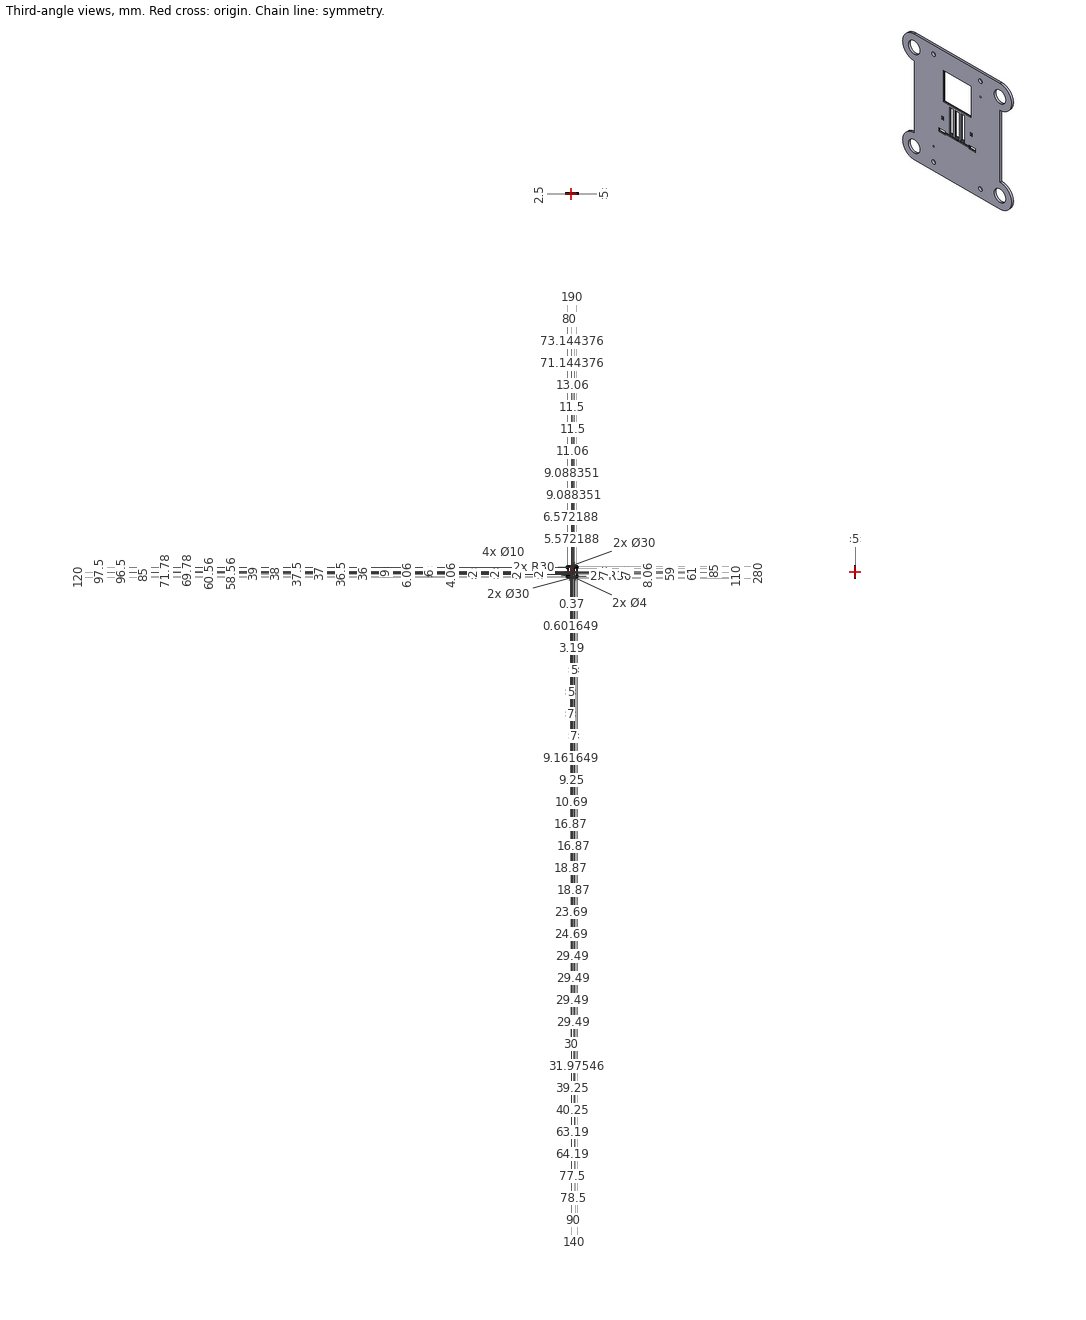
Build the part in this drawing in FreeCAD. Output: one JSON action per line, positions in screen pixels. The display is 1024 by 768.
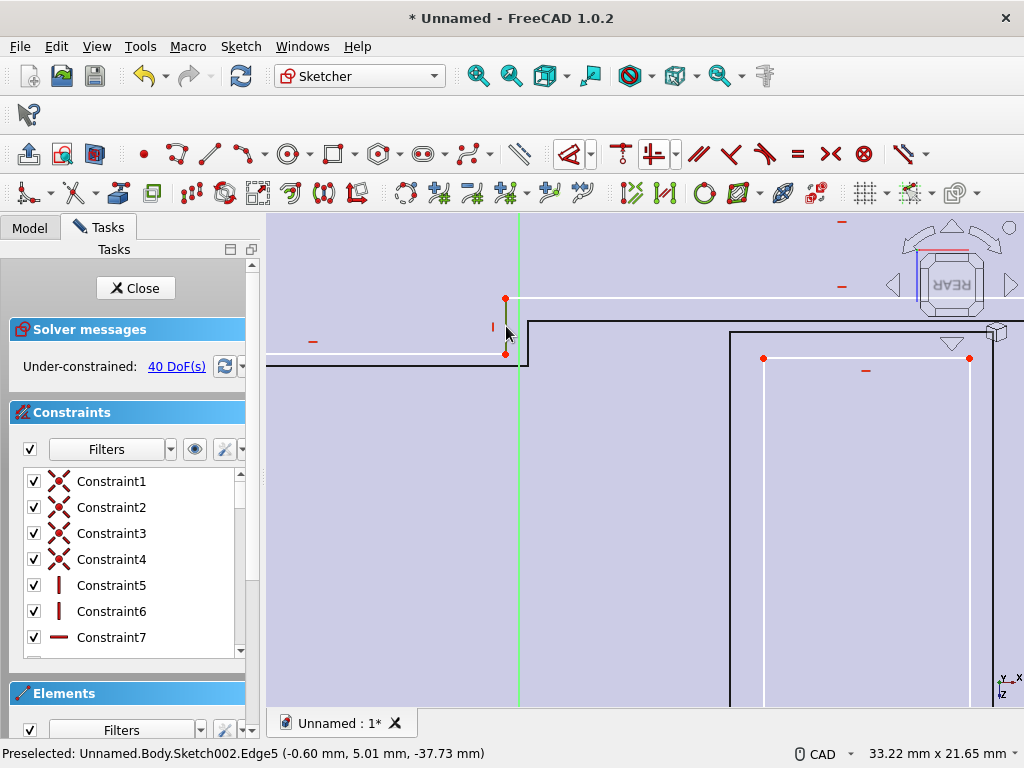
{"action": "key", "text": "i"}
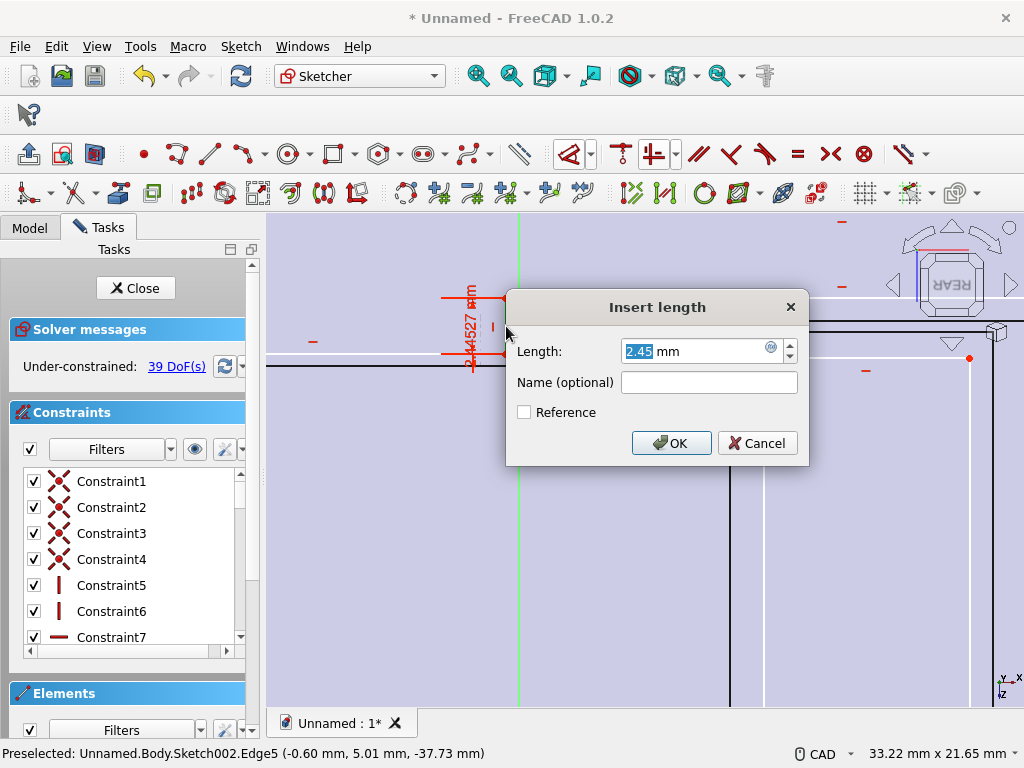
{"action": "type", "text": "2"}
{"action": "key", "text": "Return"}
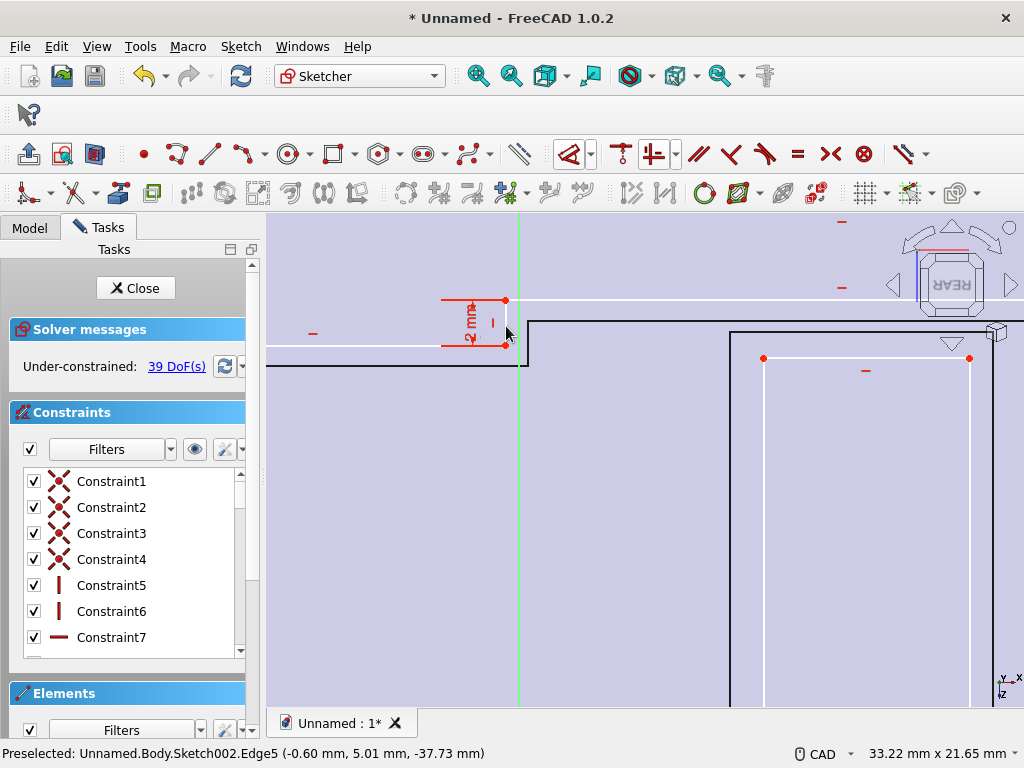
{"action": "scroll", "coordinate": [514, 329], "scroll_direction": "down", "scroll_amount": 12}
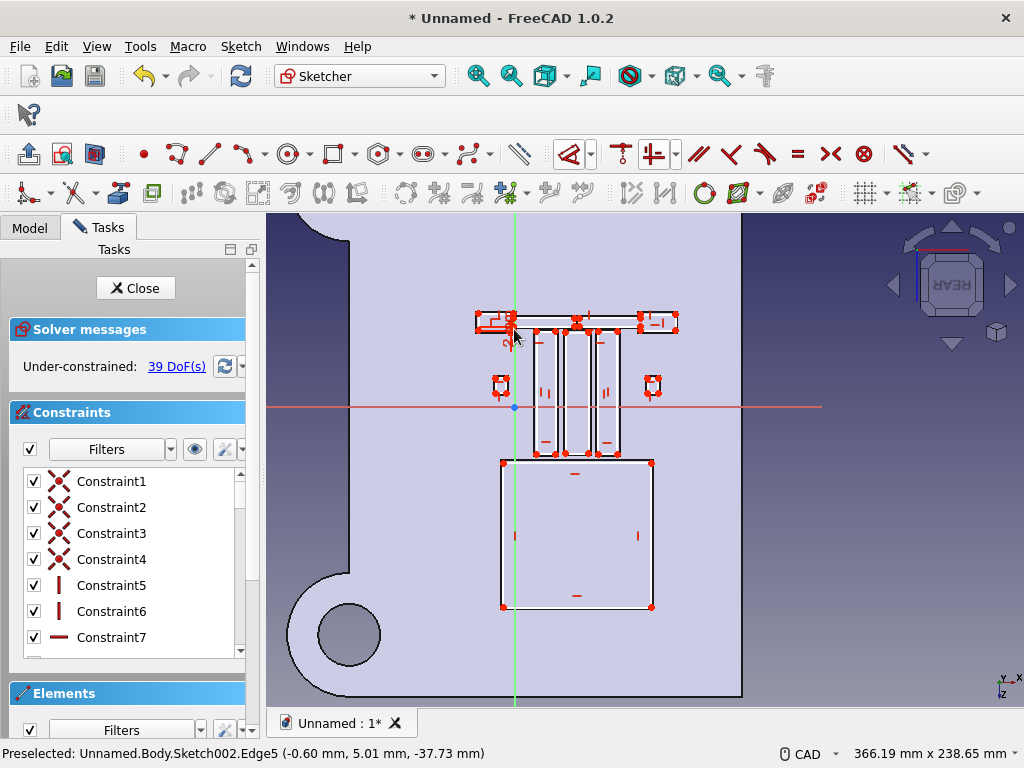
{"action": "scroll", "coordinate": [514, 317], "scroll_direction": "up", "scroll_amount": 13}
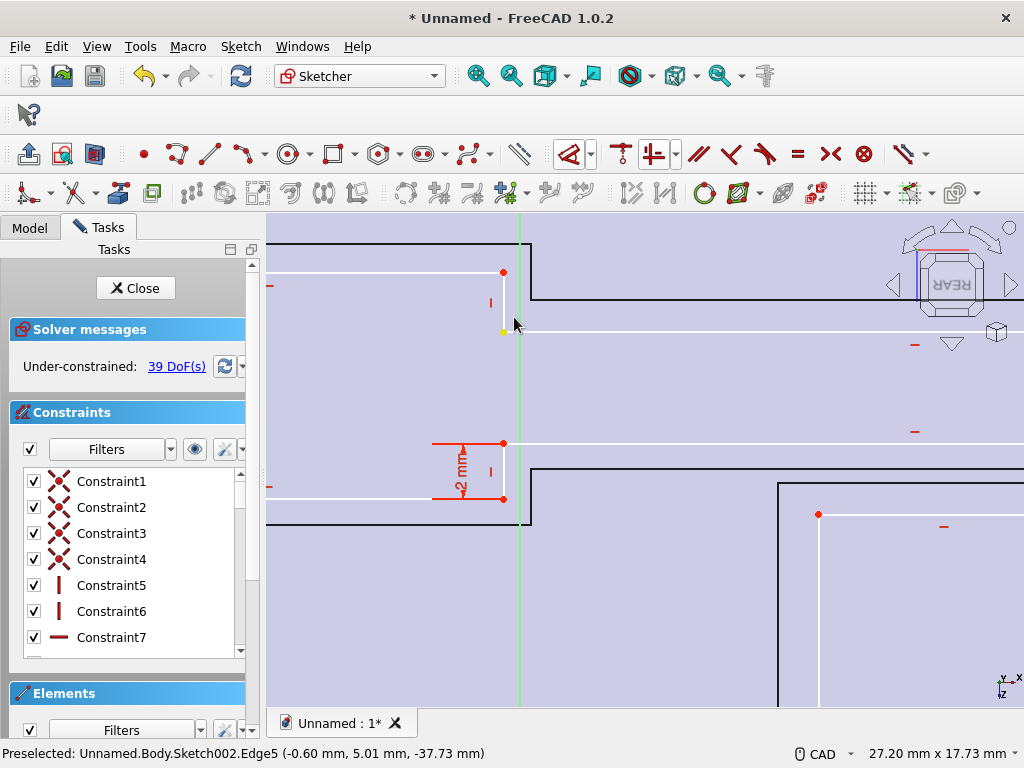
{"action": "left_click", "coordinate": [504, 314]}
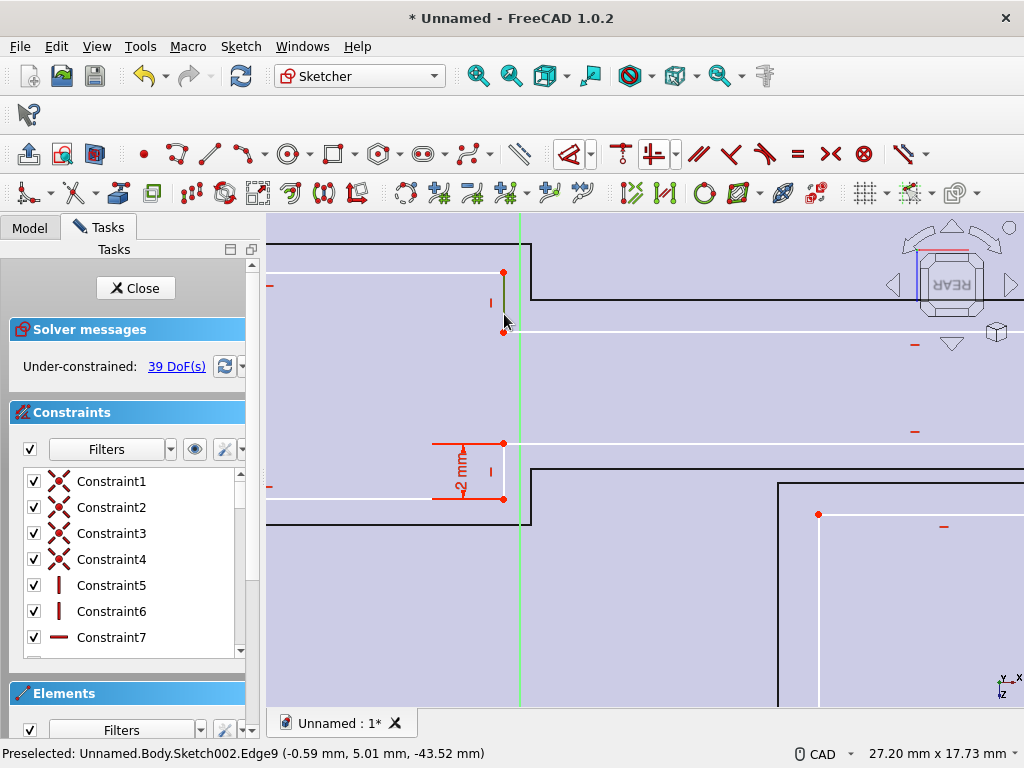
{"action": "left_click", "coordinate": [590, 154]}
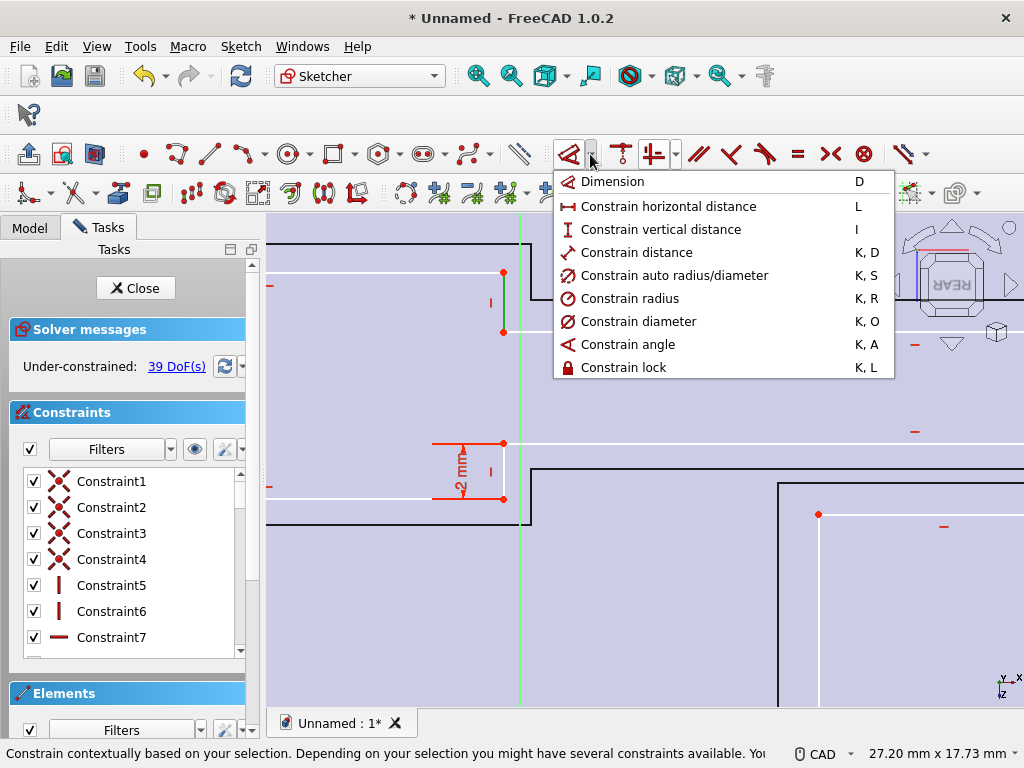
{"action": "left_click", "coordinate": [724, 230]}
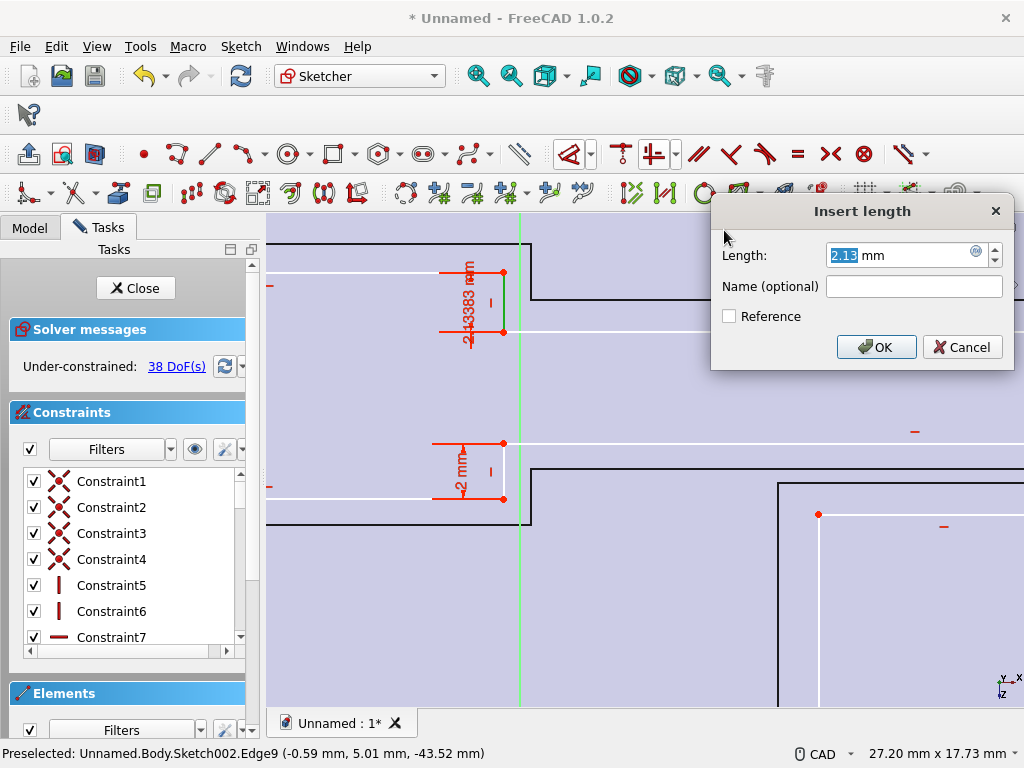
{"action": "type", "text": "2"}
{"action": "key", "text": "Return"}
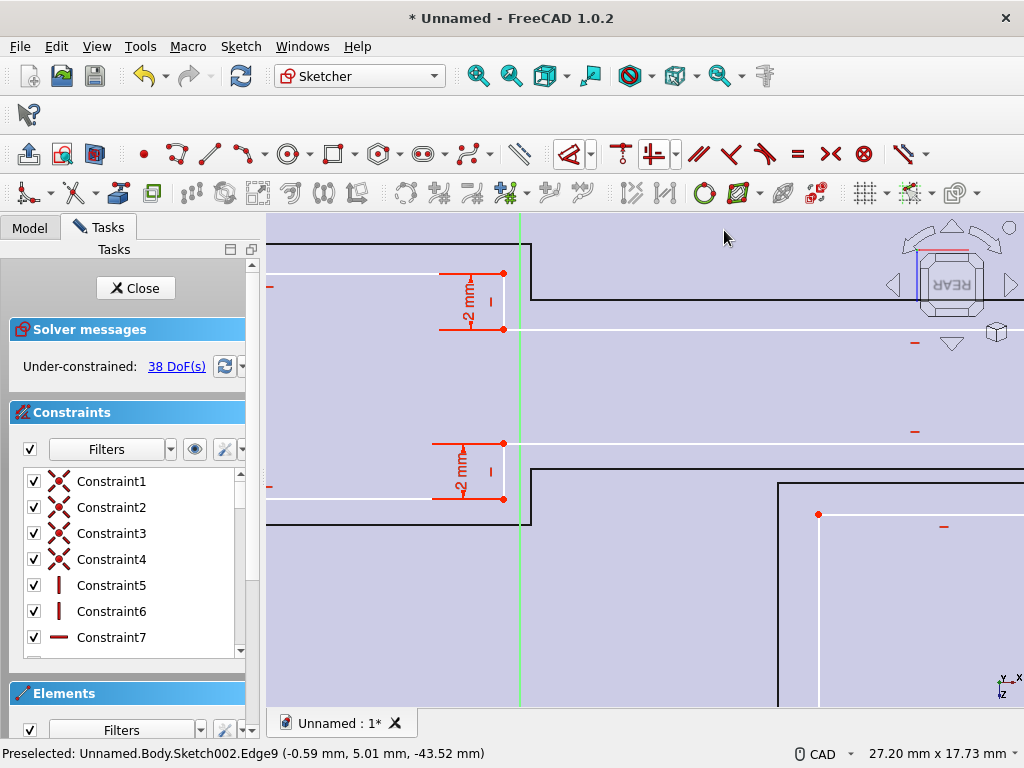
{"action": "scroll", "coordinate": [514, 317], "scroll_direction": "down", "scroll_amount": 13}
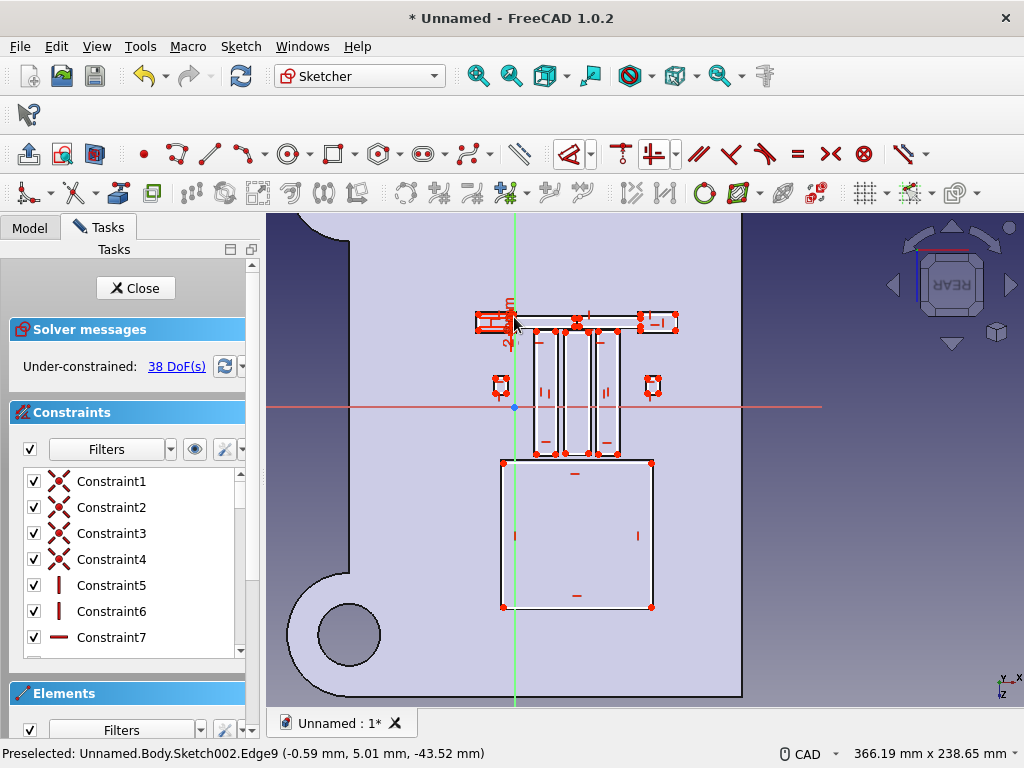
{"action": "scroll", "coordinate": [640, 328], "scroll_direction": "up", "scroll_amount": 13}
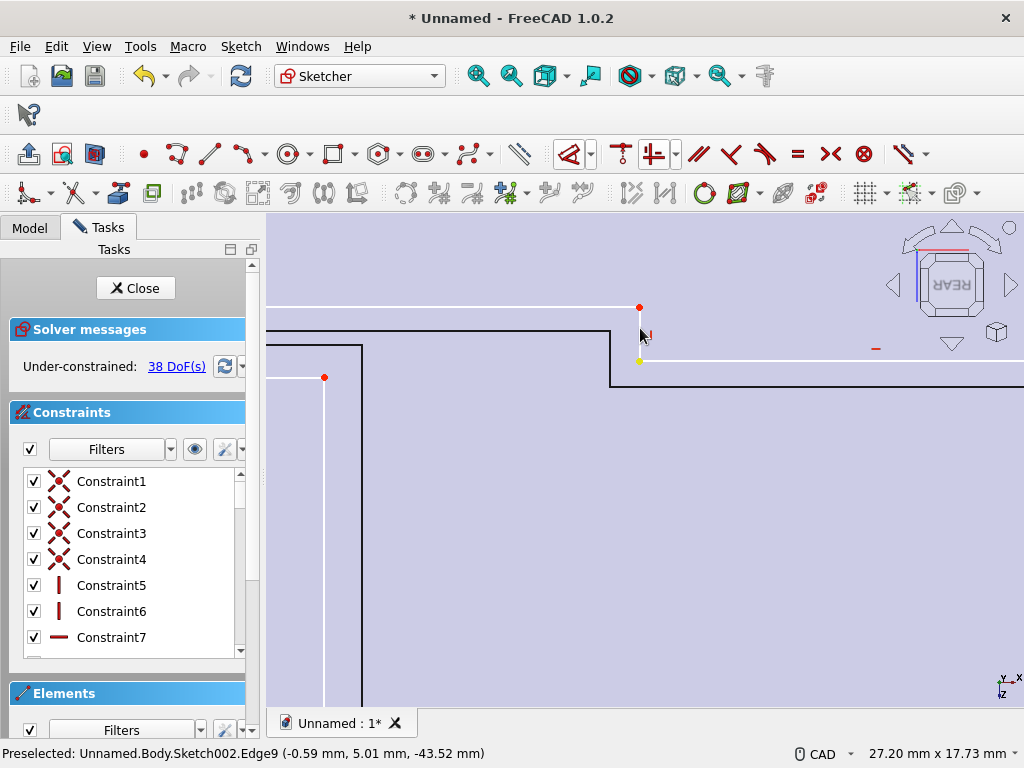
{"action": "left_click", "coordinate": [640, 323]}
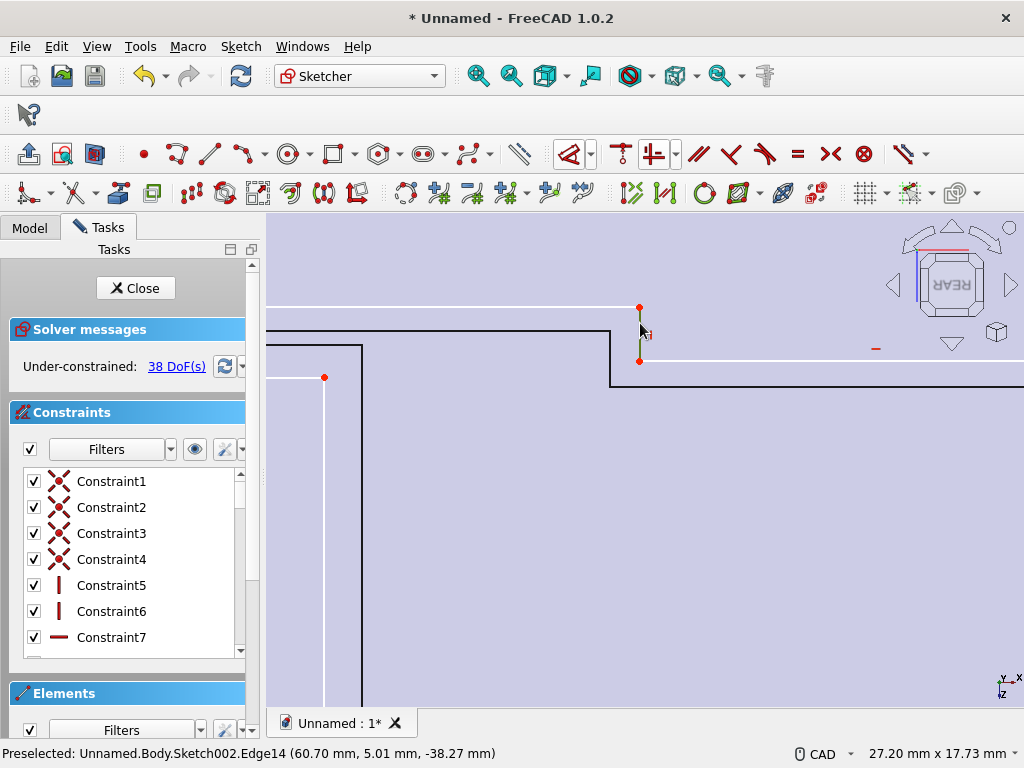
{"action": "left_click", "coordinate": [590, 154]}